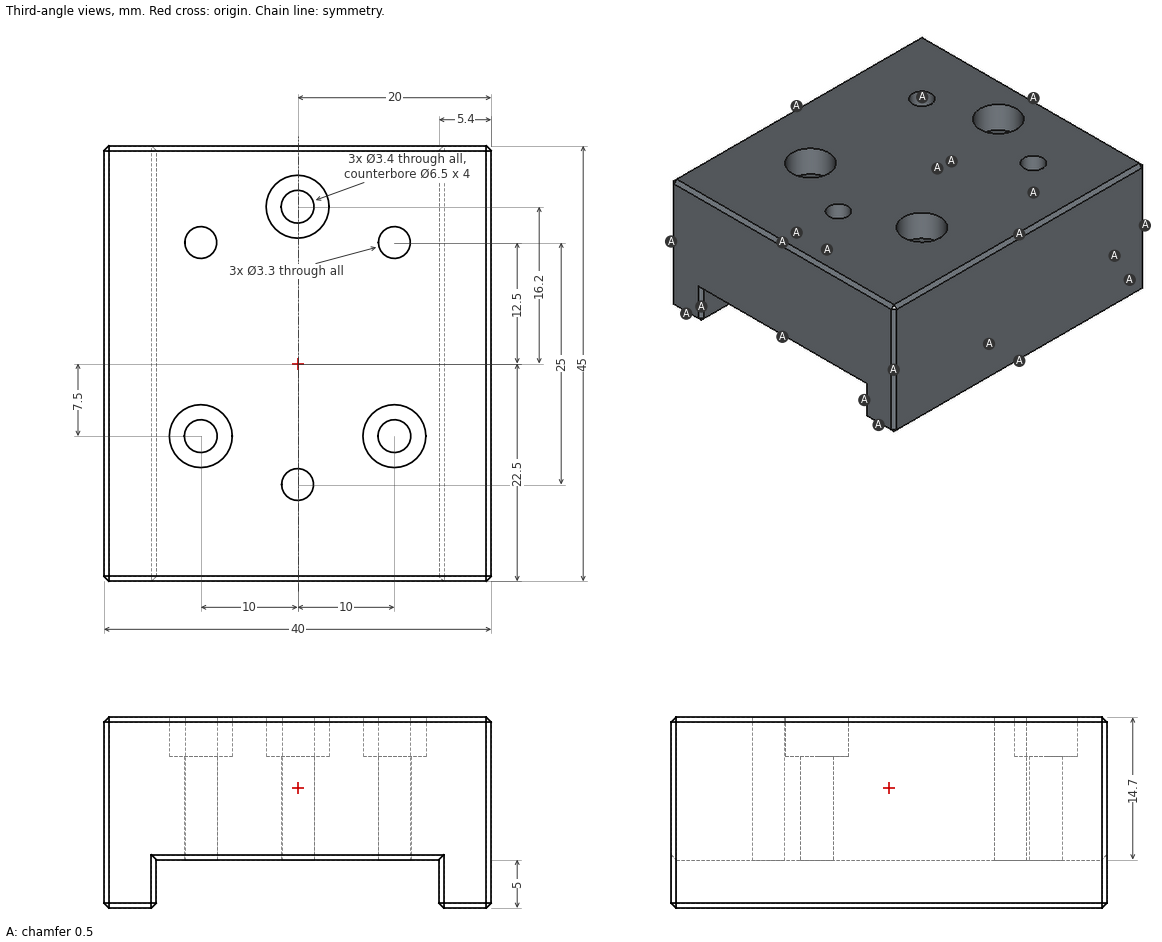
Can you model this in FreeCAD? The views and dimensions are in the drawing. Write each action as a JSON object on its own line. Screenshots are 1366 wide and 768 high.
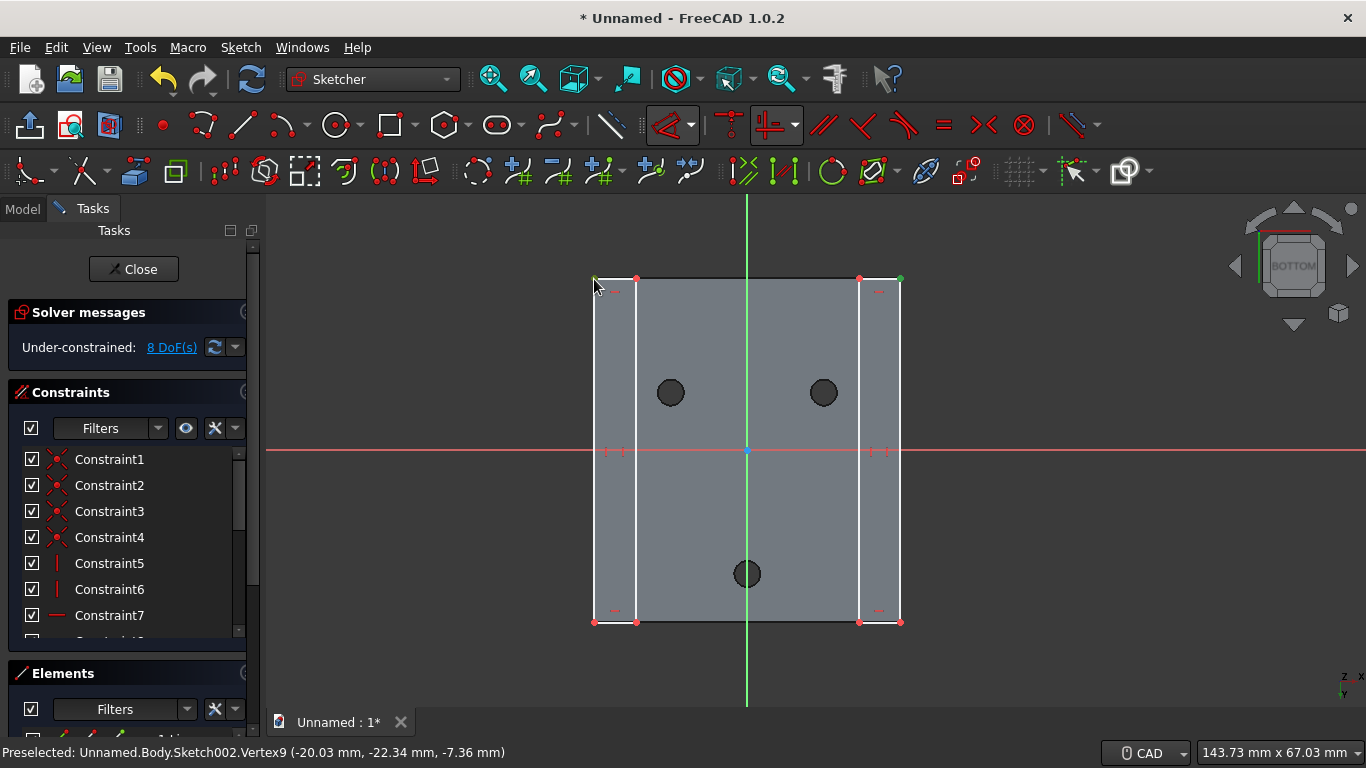
{"action": "left_click", "coordinate": [747, 646]}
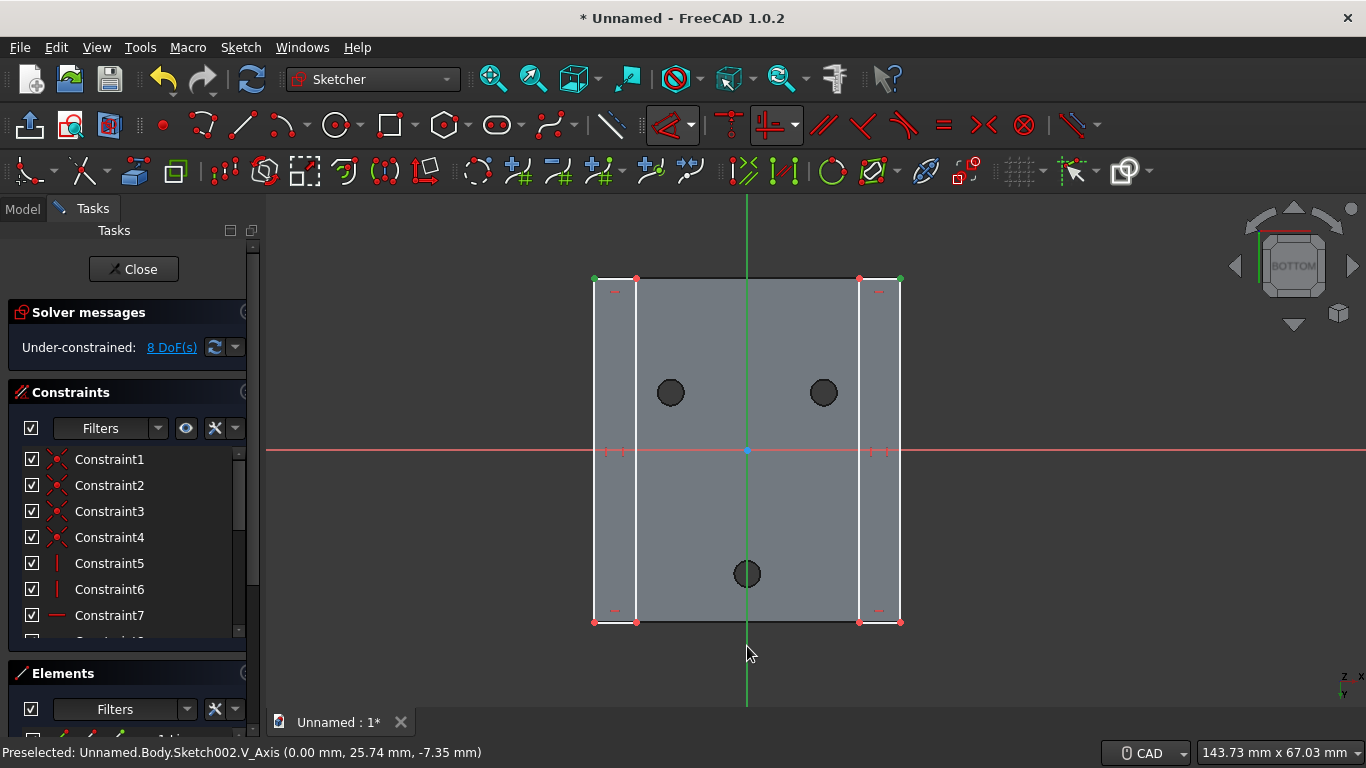
{"action": "left_click", "coordinate": [984, 126]}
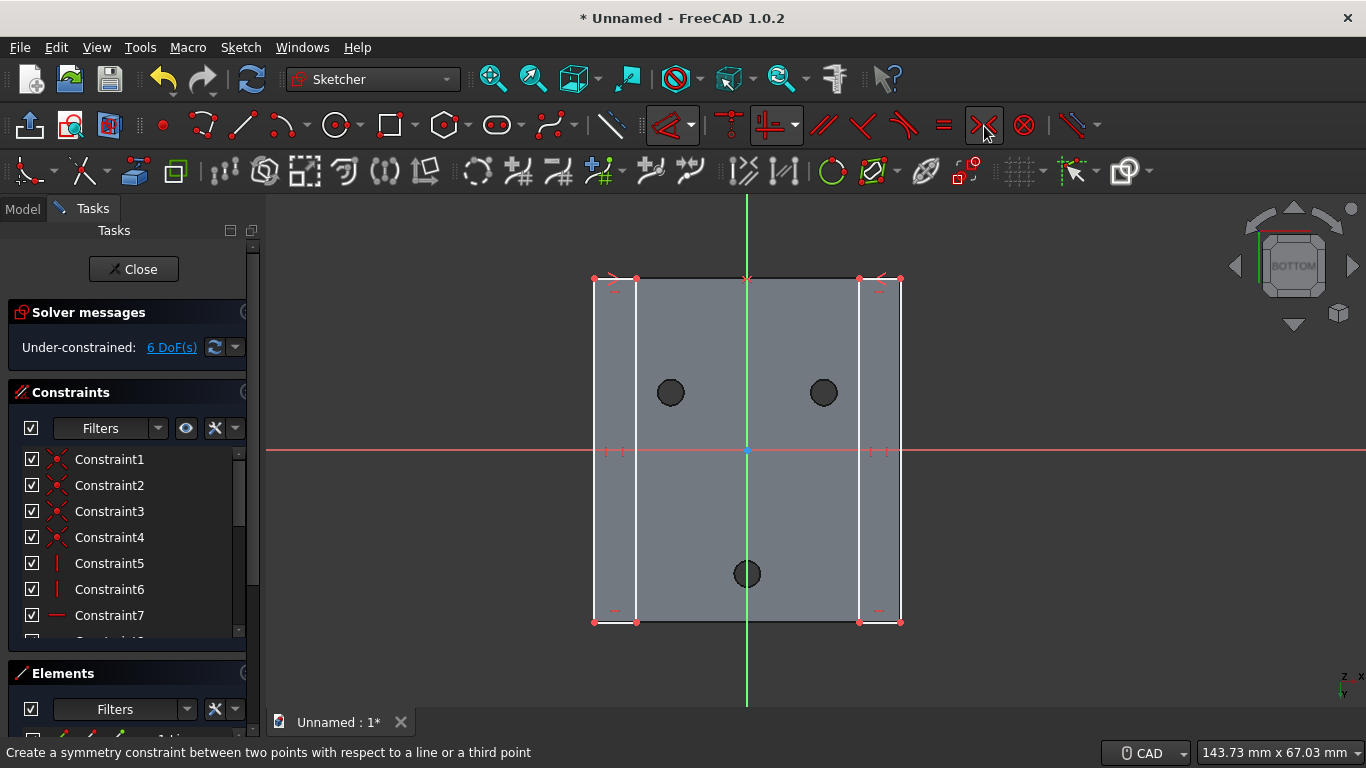
{"action": "left_click", "coordinate": [859, 623]}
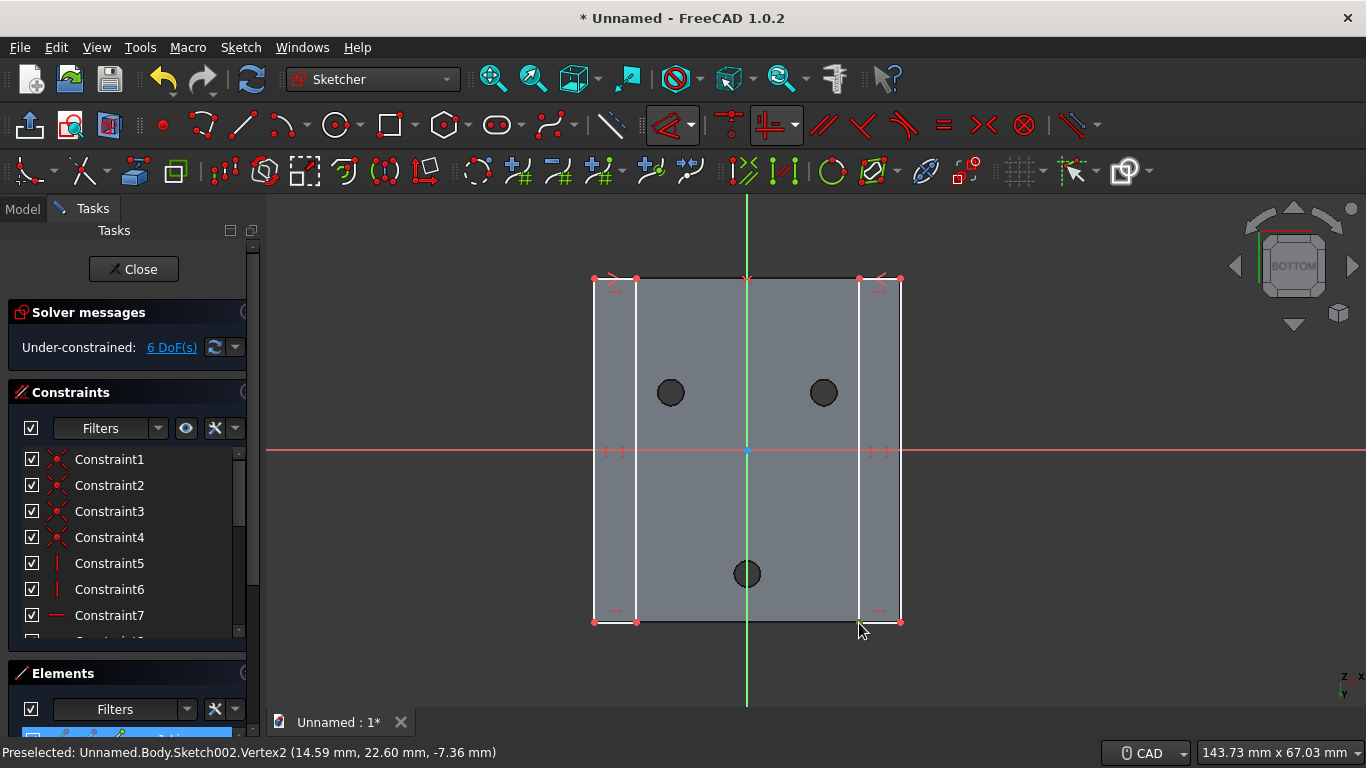
{"action": "left_click", "coordinate": [636, 623]}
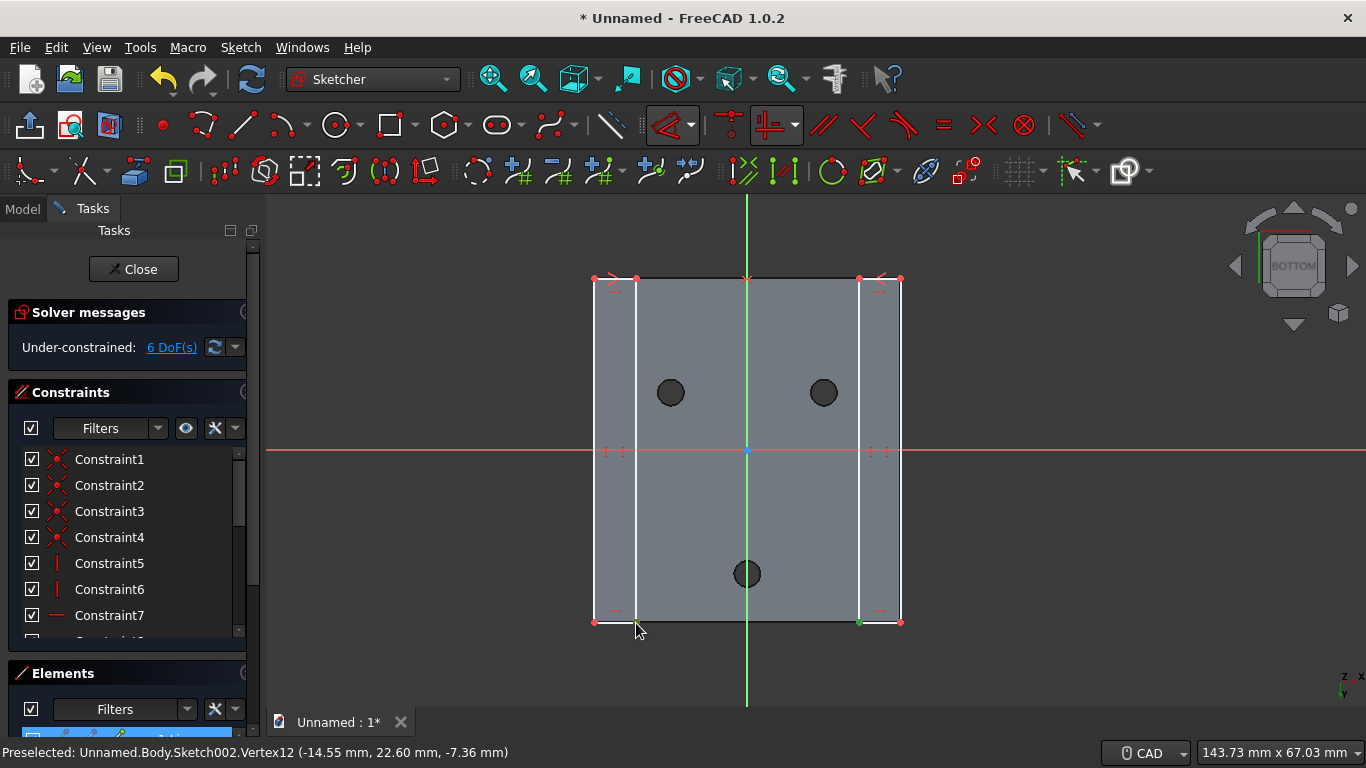
{"action": "left_click", "coordinate": [747, 646]}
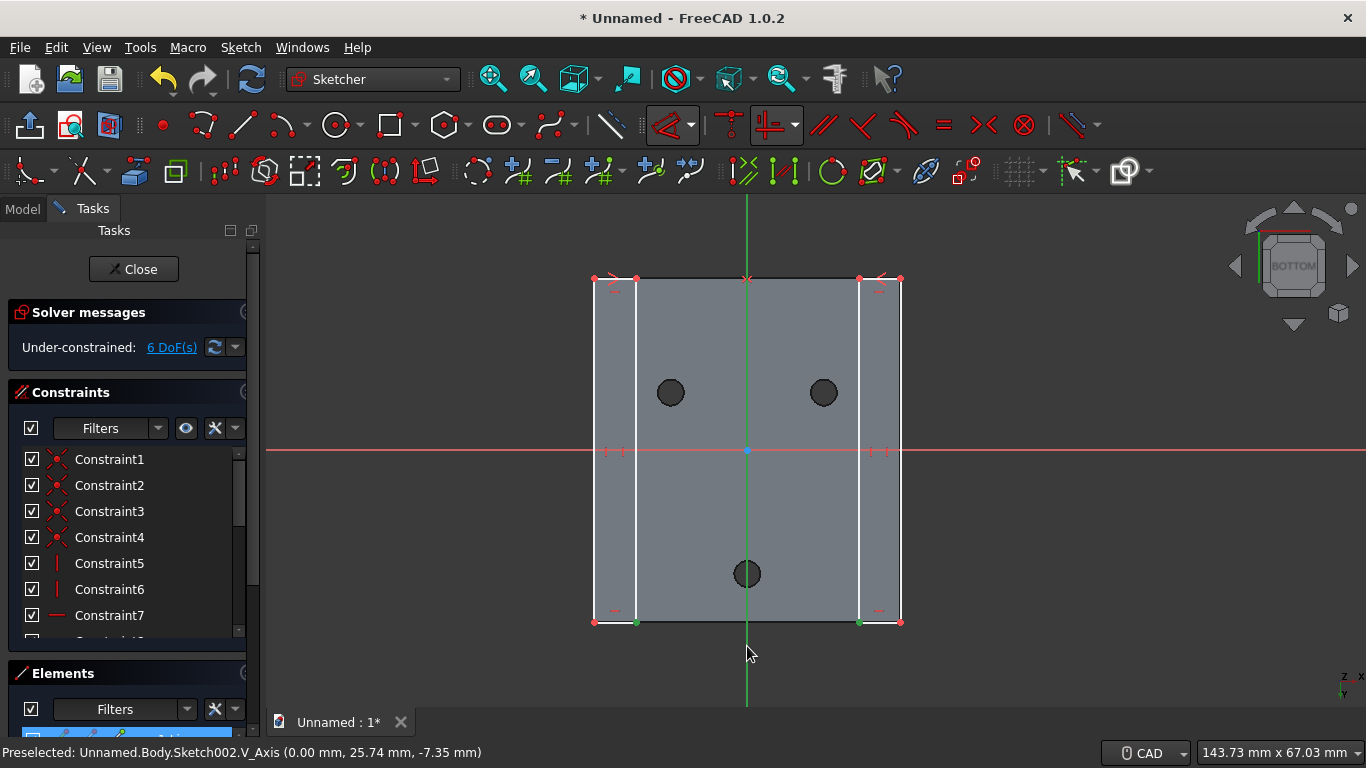
{"action": "left_click", "coordinate": [984, 126]}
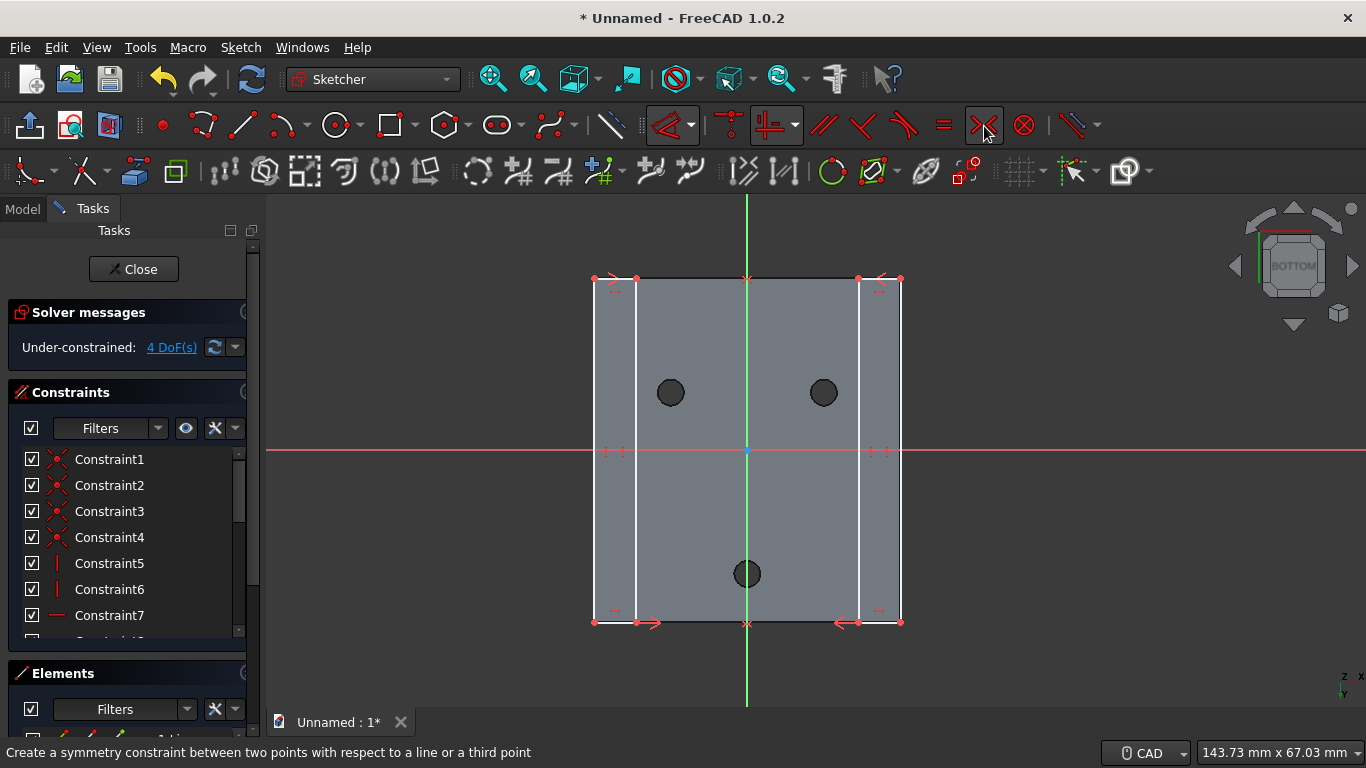
{"action": "left_click", "coordinate": [859, 382]}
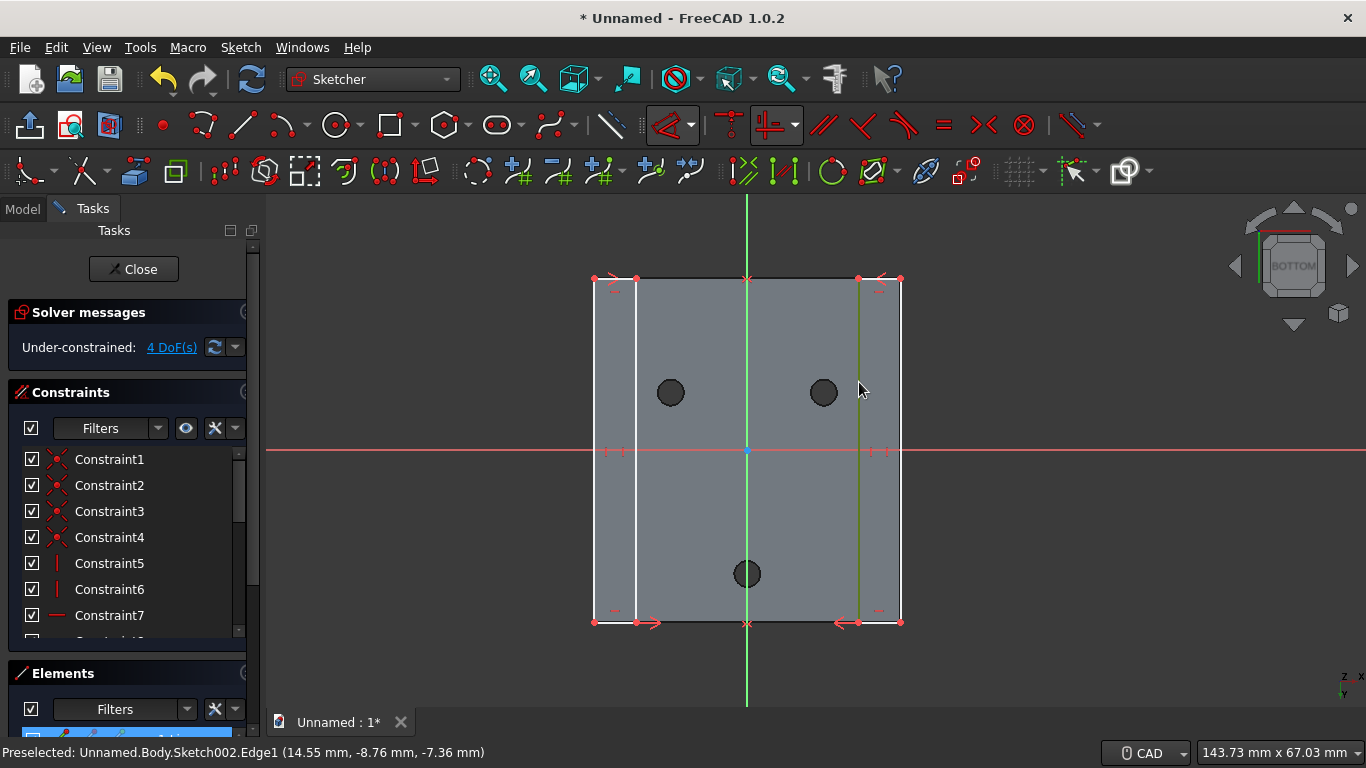
{"action": "key", "text": "i"}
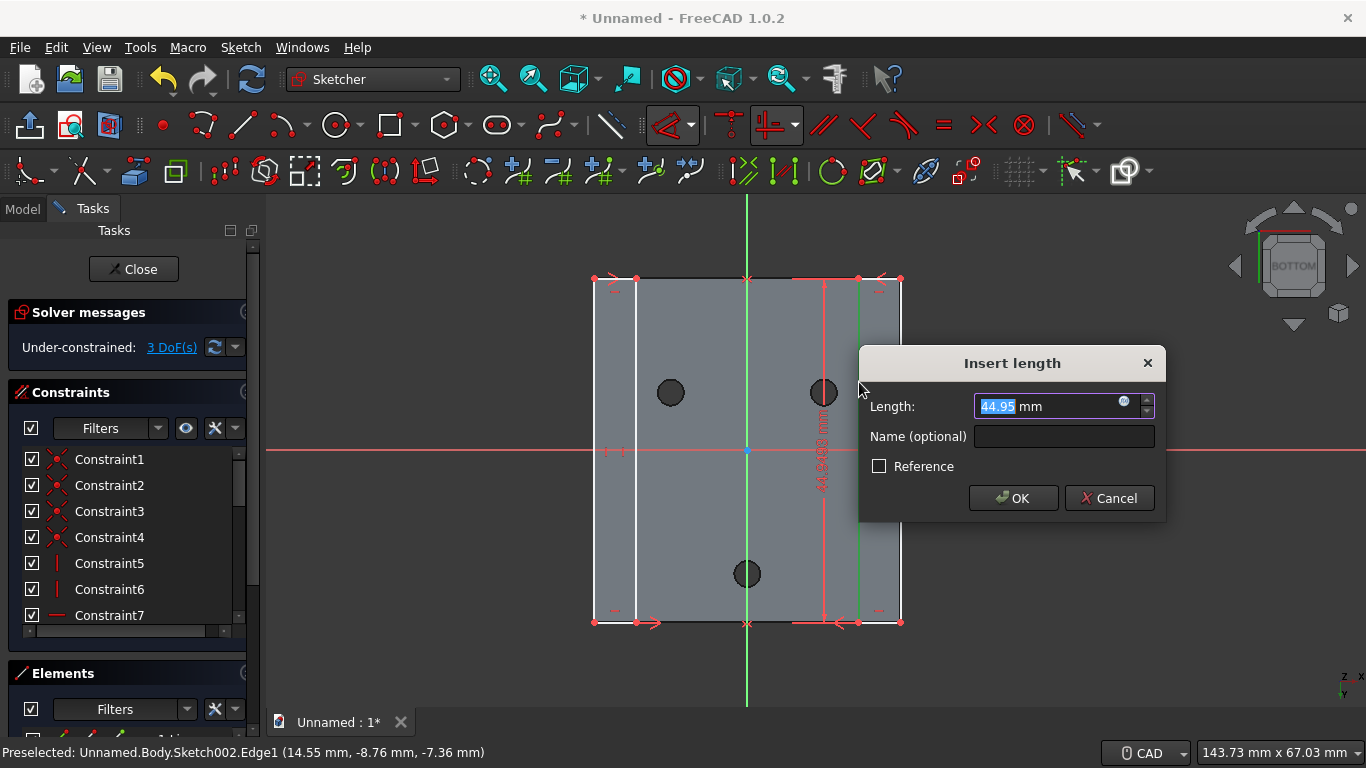
{"action": "type", "text": "45"}
{"action": "key", "text": "Return"}